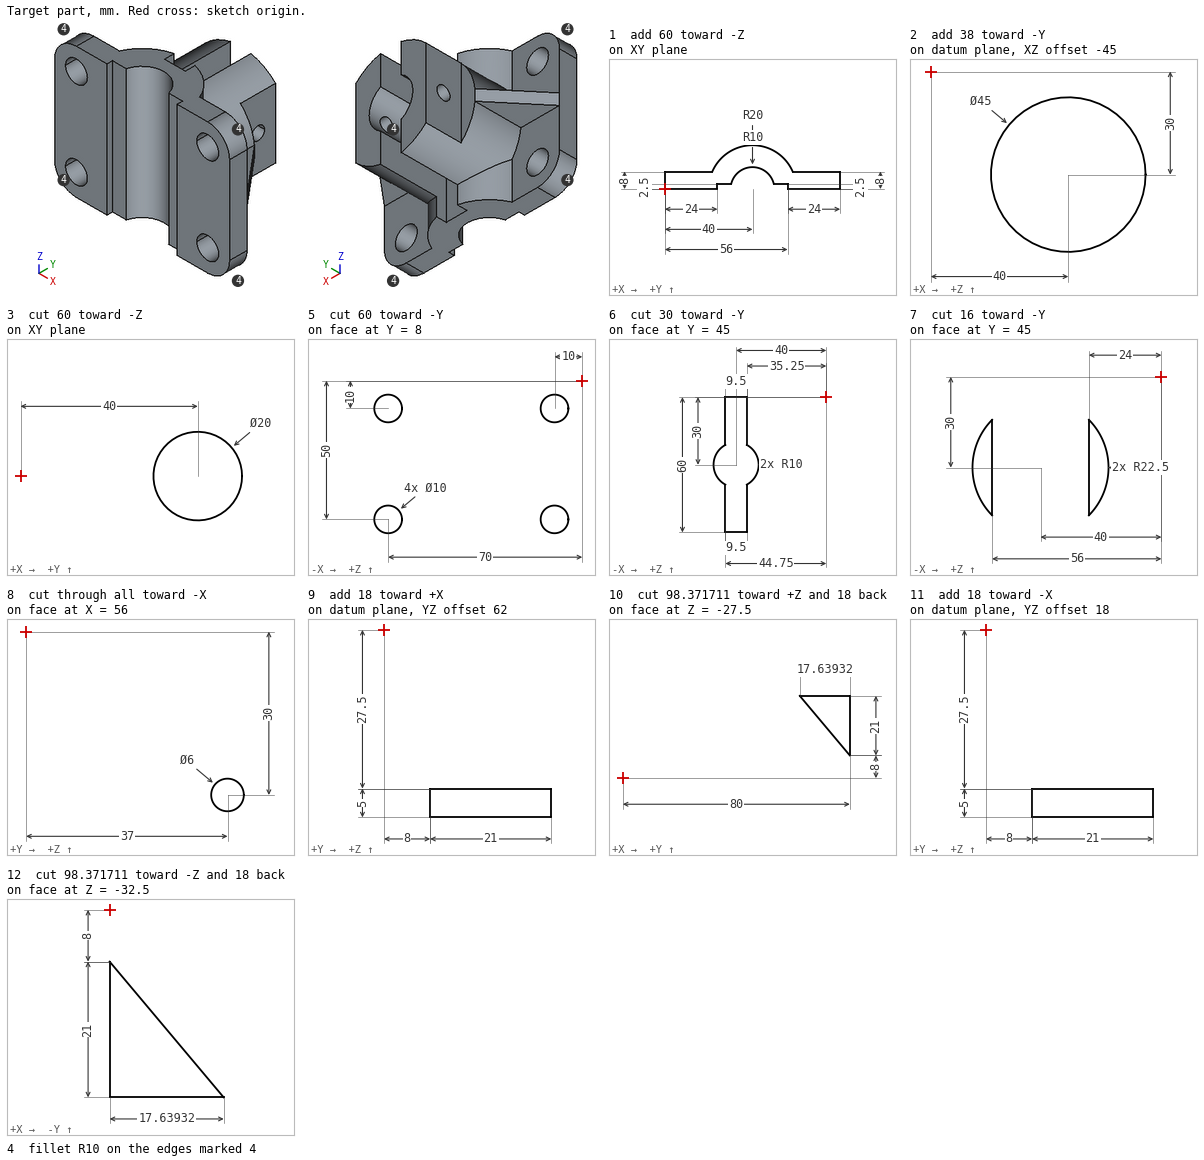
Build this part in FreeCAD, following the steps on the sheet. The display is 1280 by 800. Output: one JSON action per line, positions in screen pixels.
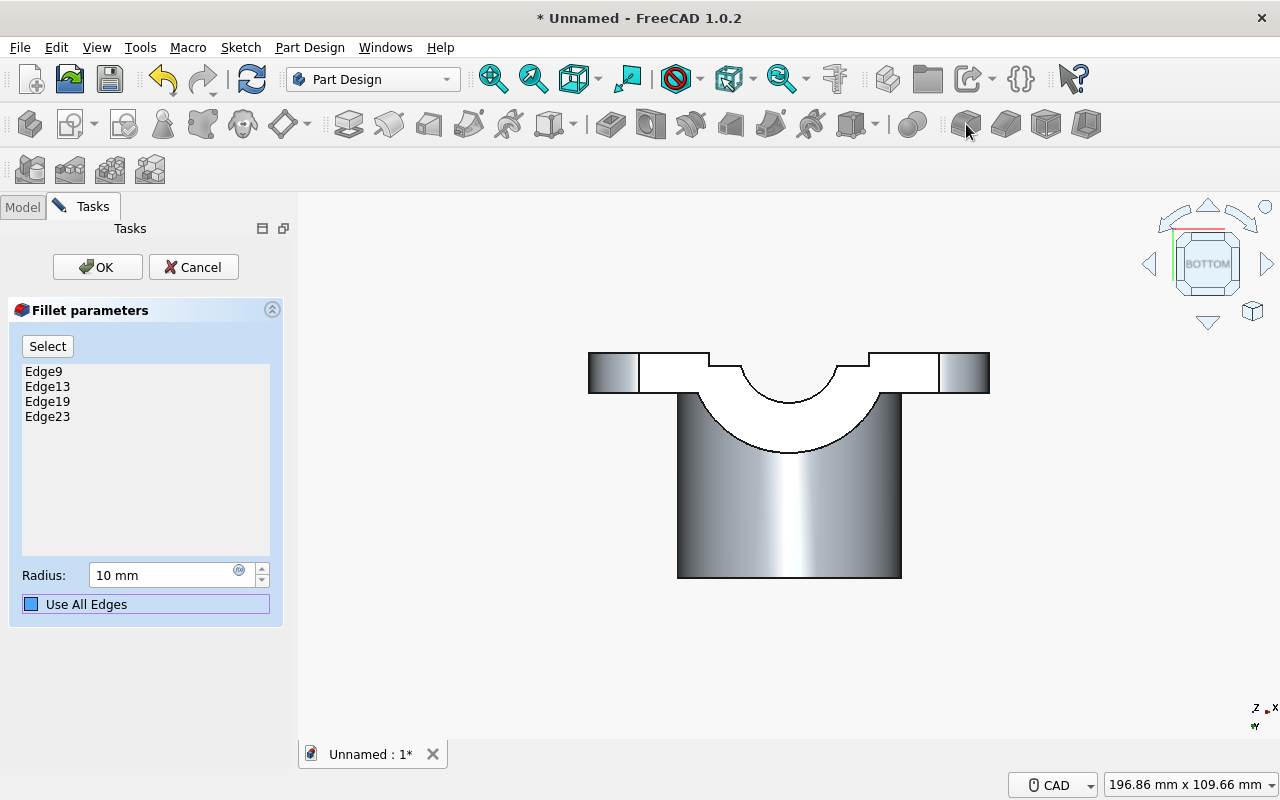
{"action": "left_click", "coordinate": [98, 267]}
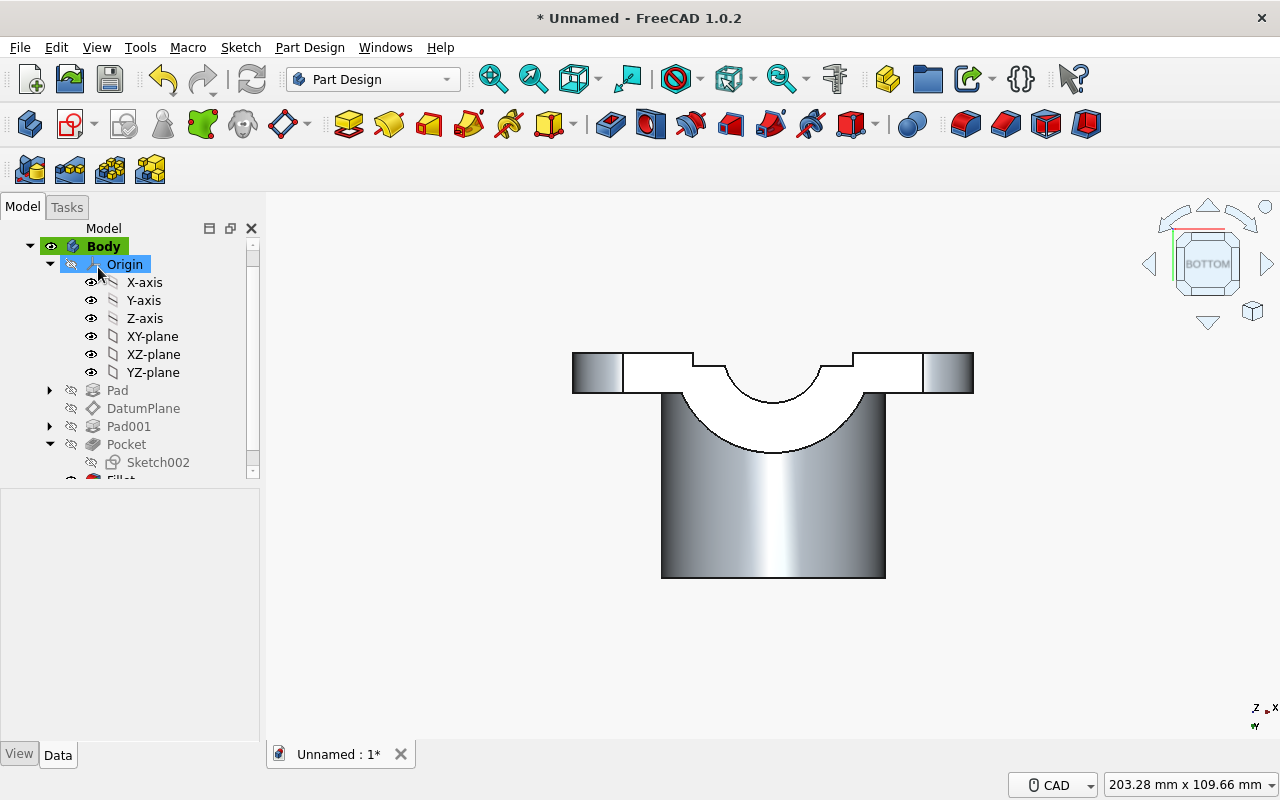
{"action": "left_click", "coordinate": [494, 80]}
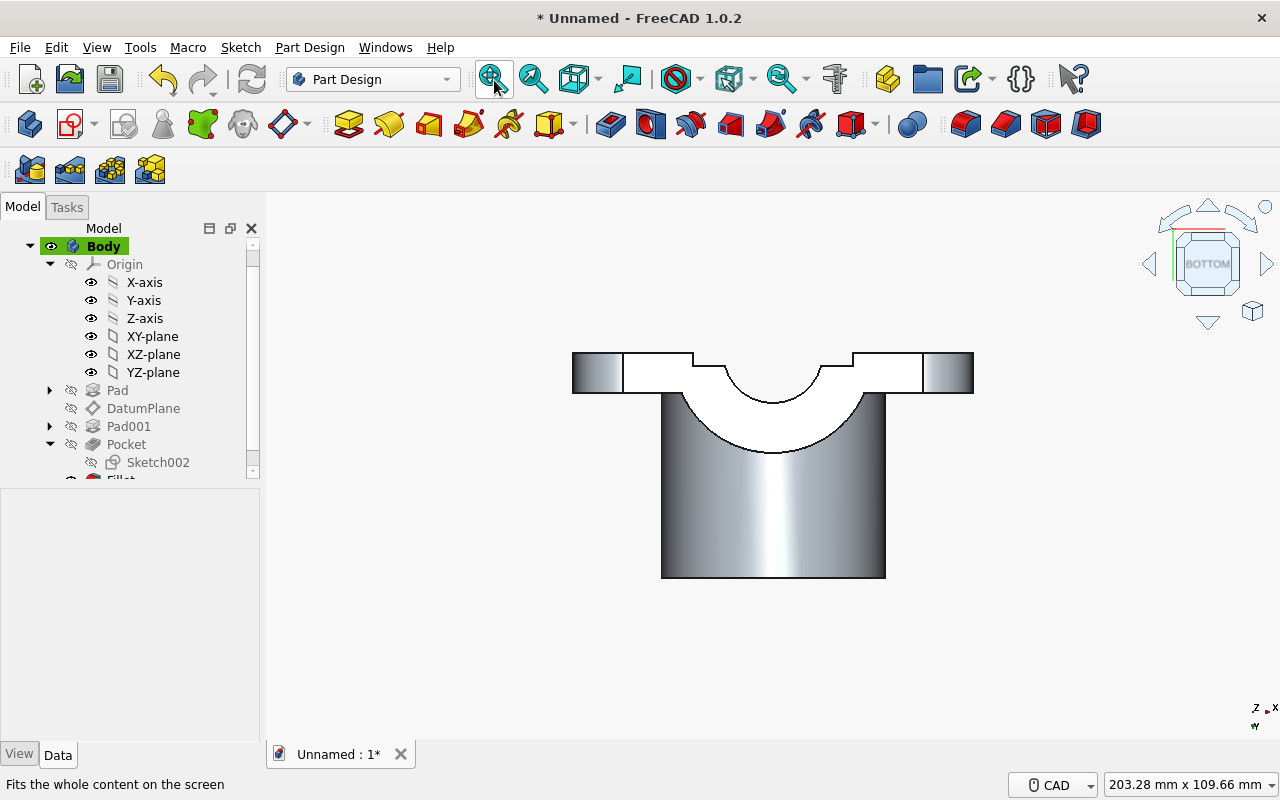
{"action": "key", "text": "4"}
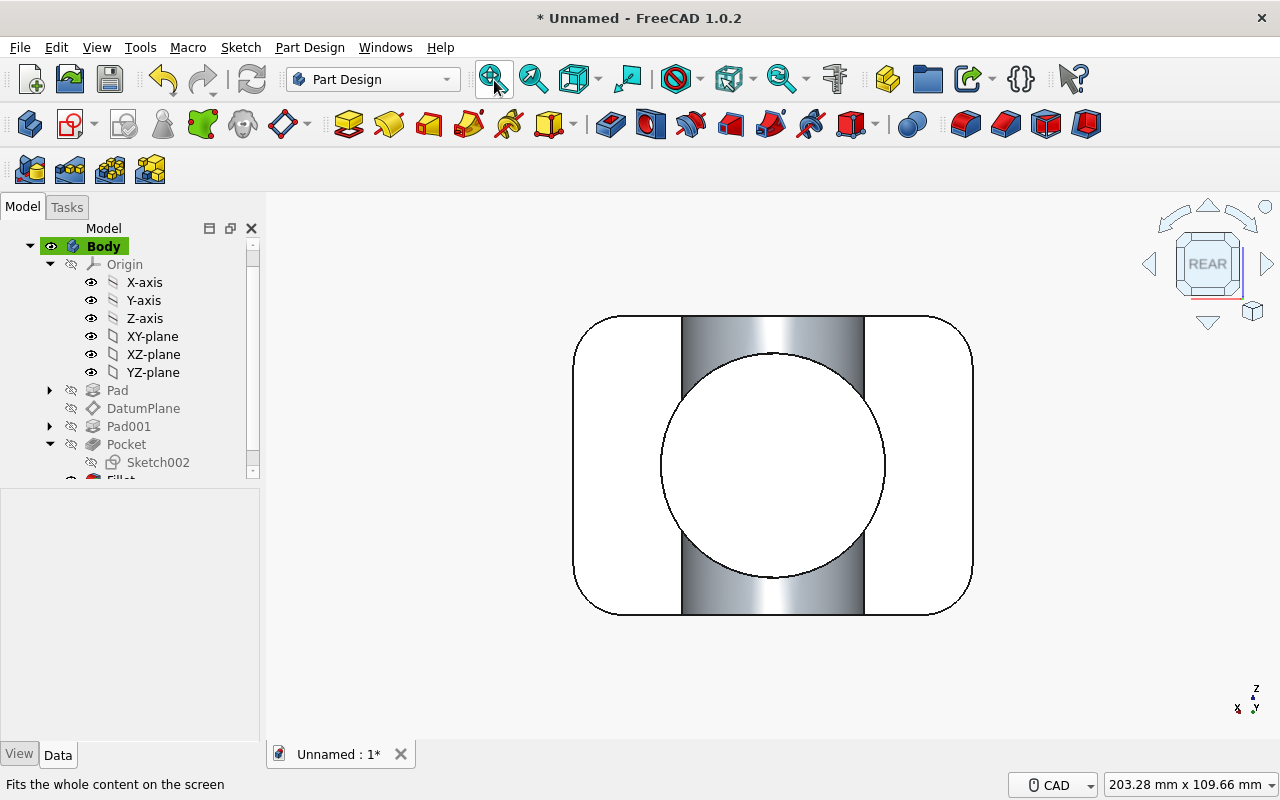
{"action": "left_click", "coordinate": [628, 379]}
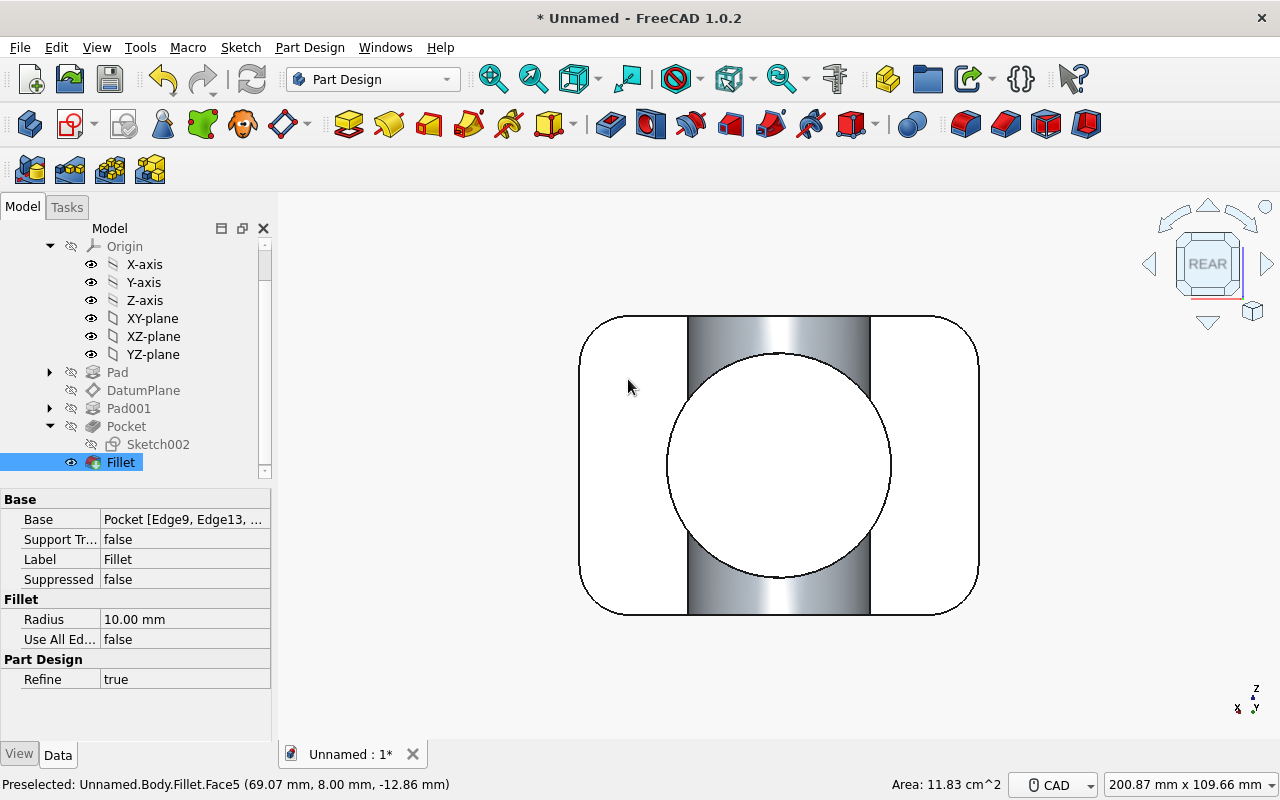
{"action": "left_click", "coordinate": [70, 124]}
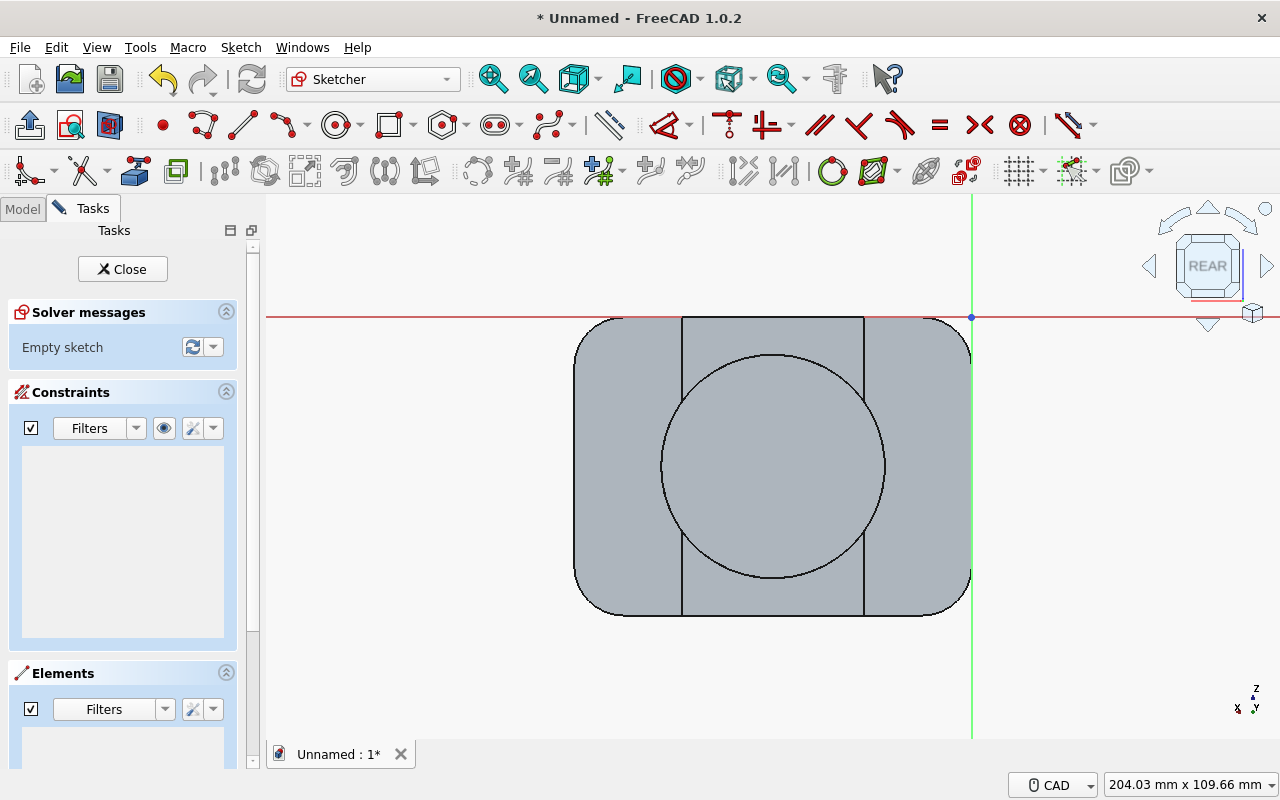
{"action": "left_click", "coordinate": [336, 126]}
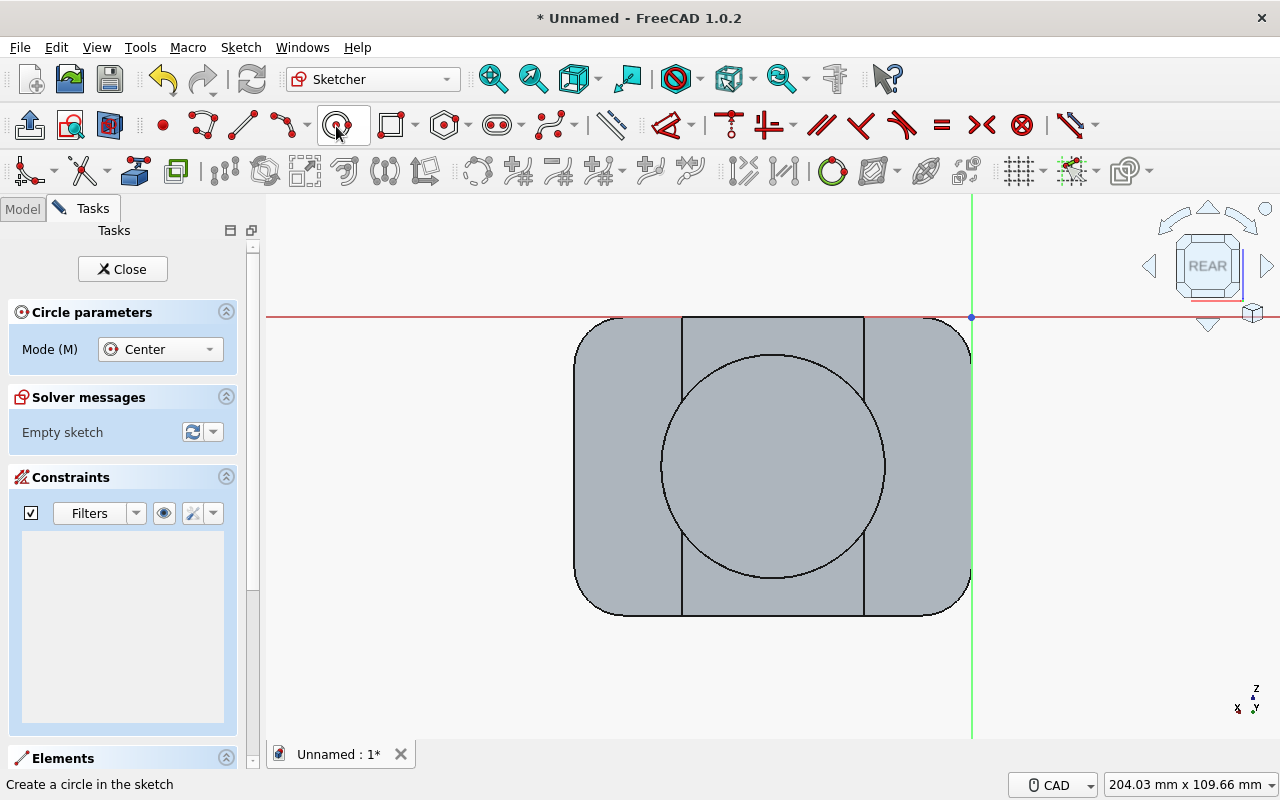
{"action": "left_click", "coordinate": [624, 566]}
{"action": "left_click", "coordinate": [641, 548]}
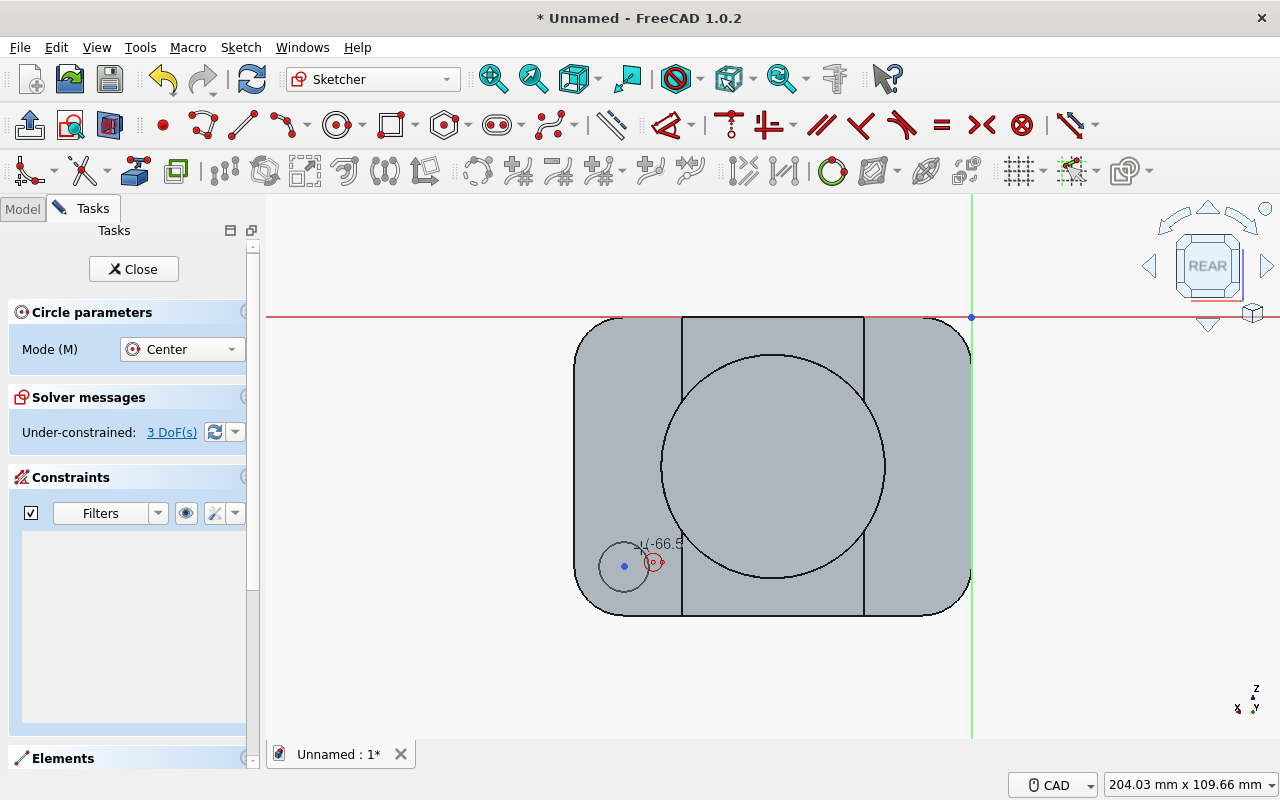
{"action": "left_click", "coordinate": [624, 367]}
{"action": "left_click", "coordinate": [641, 350]}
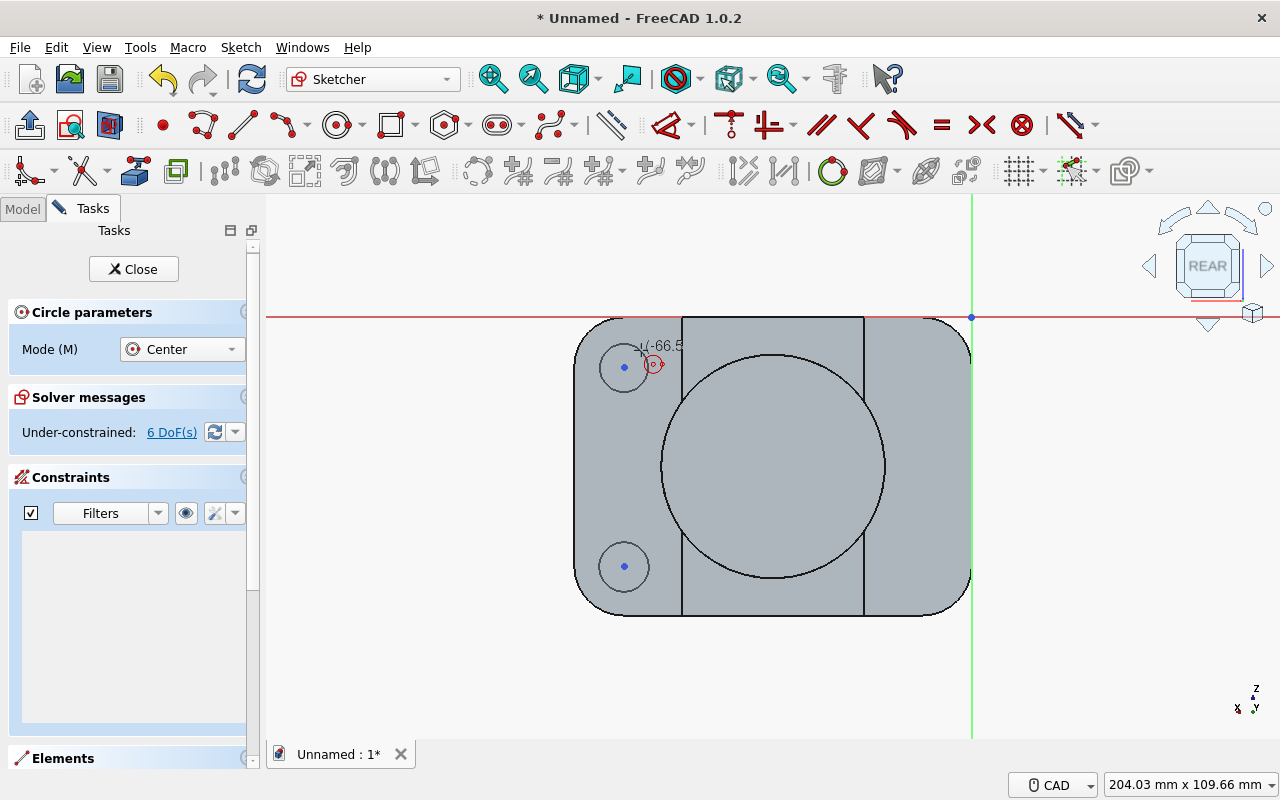
{"action": "left_click", "coordinate": [922, 367]}
{"action": "left_click", "coordinate": [940, 350]}